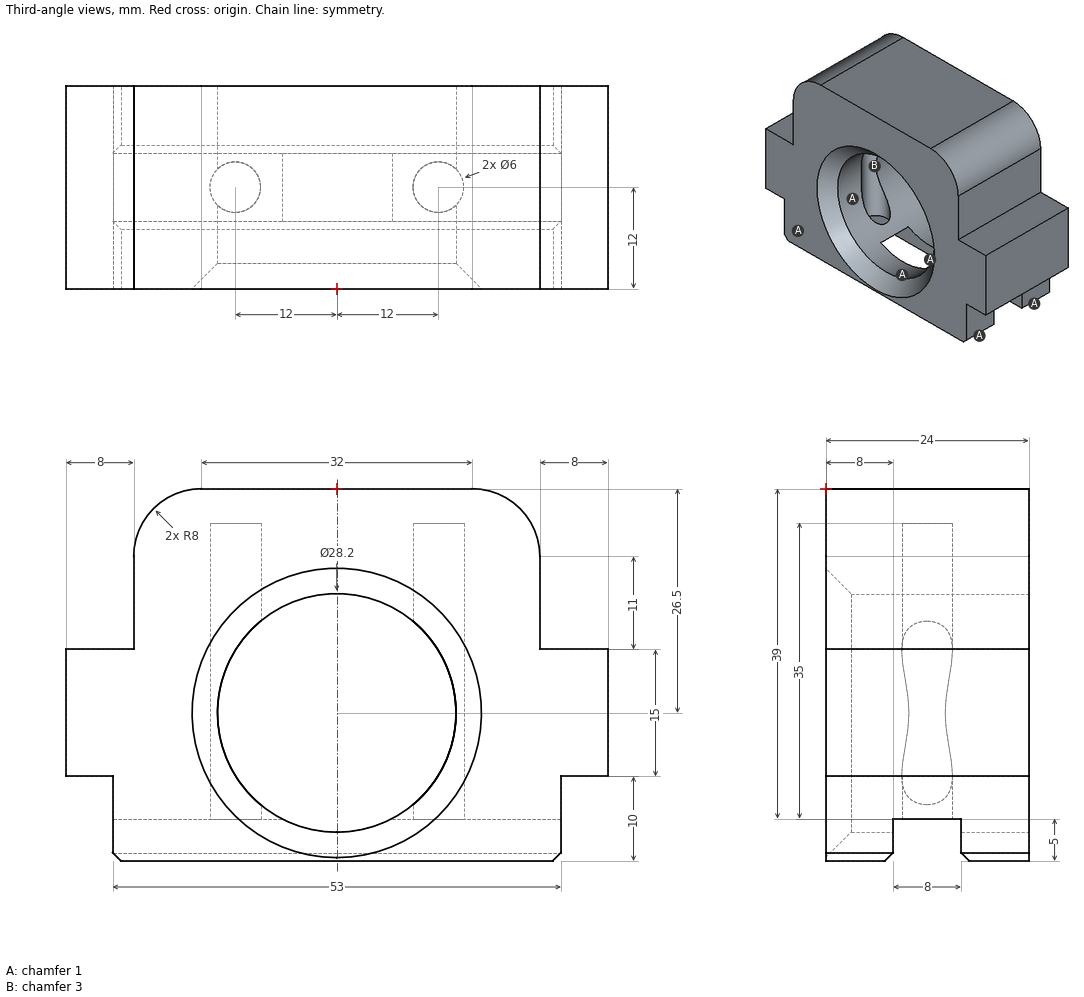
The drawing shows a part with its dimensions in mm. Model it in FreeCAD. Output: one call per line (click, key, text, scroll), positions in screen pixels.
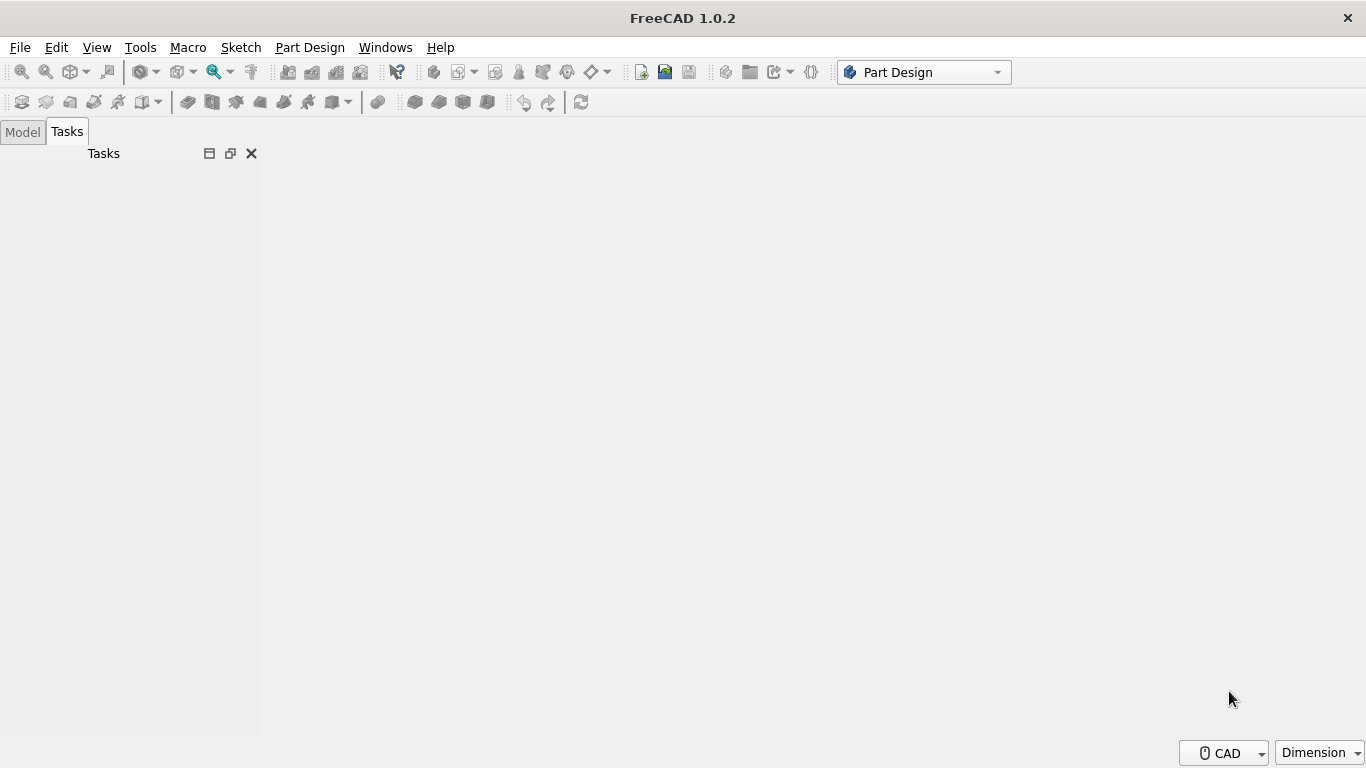
click(642, 72)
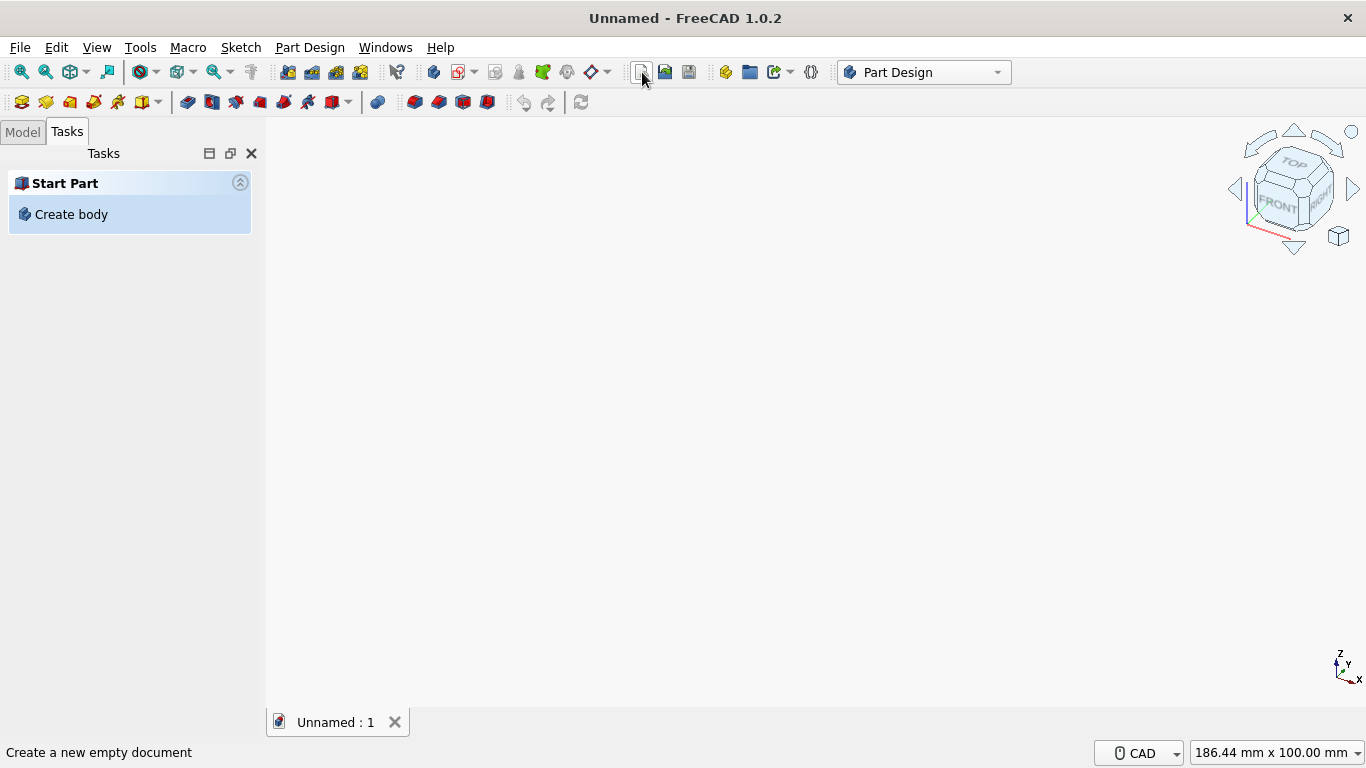
click(458, 72)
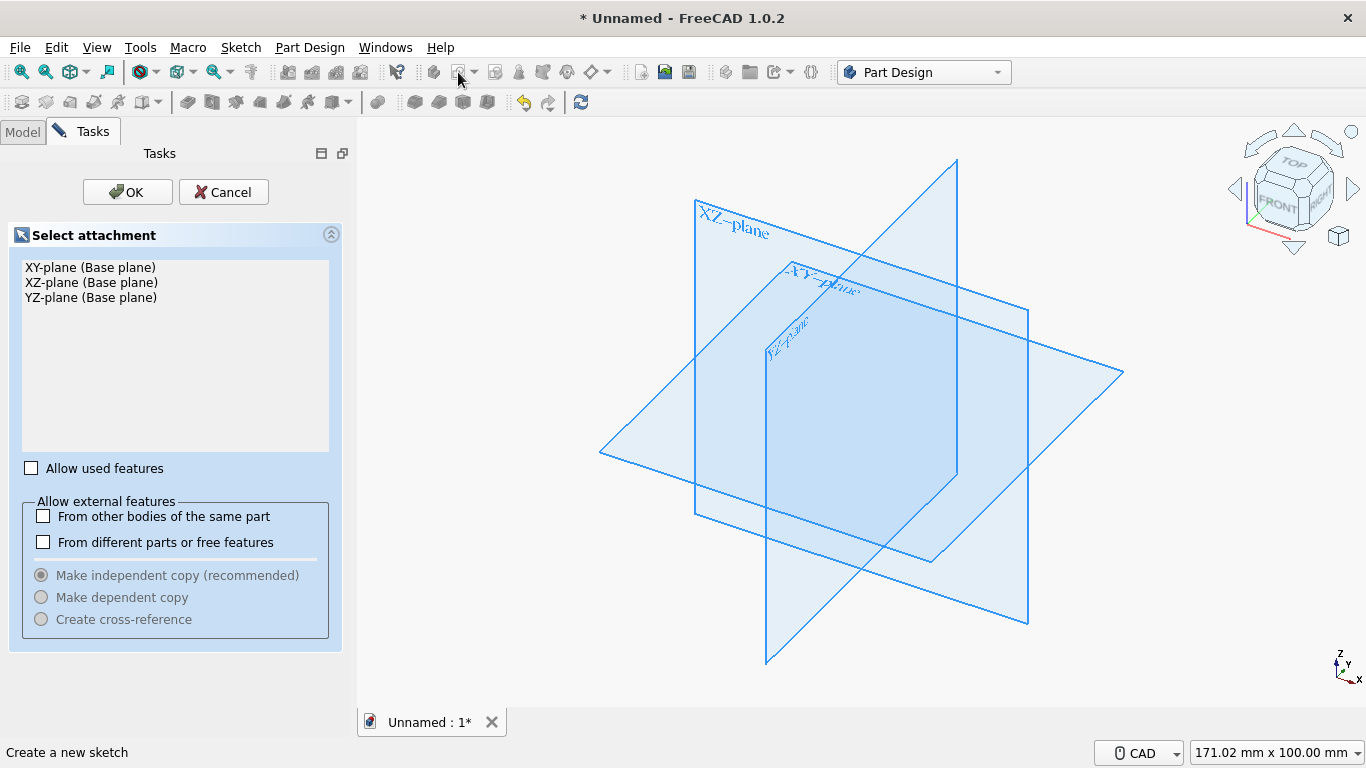
click(82, 282)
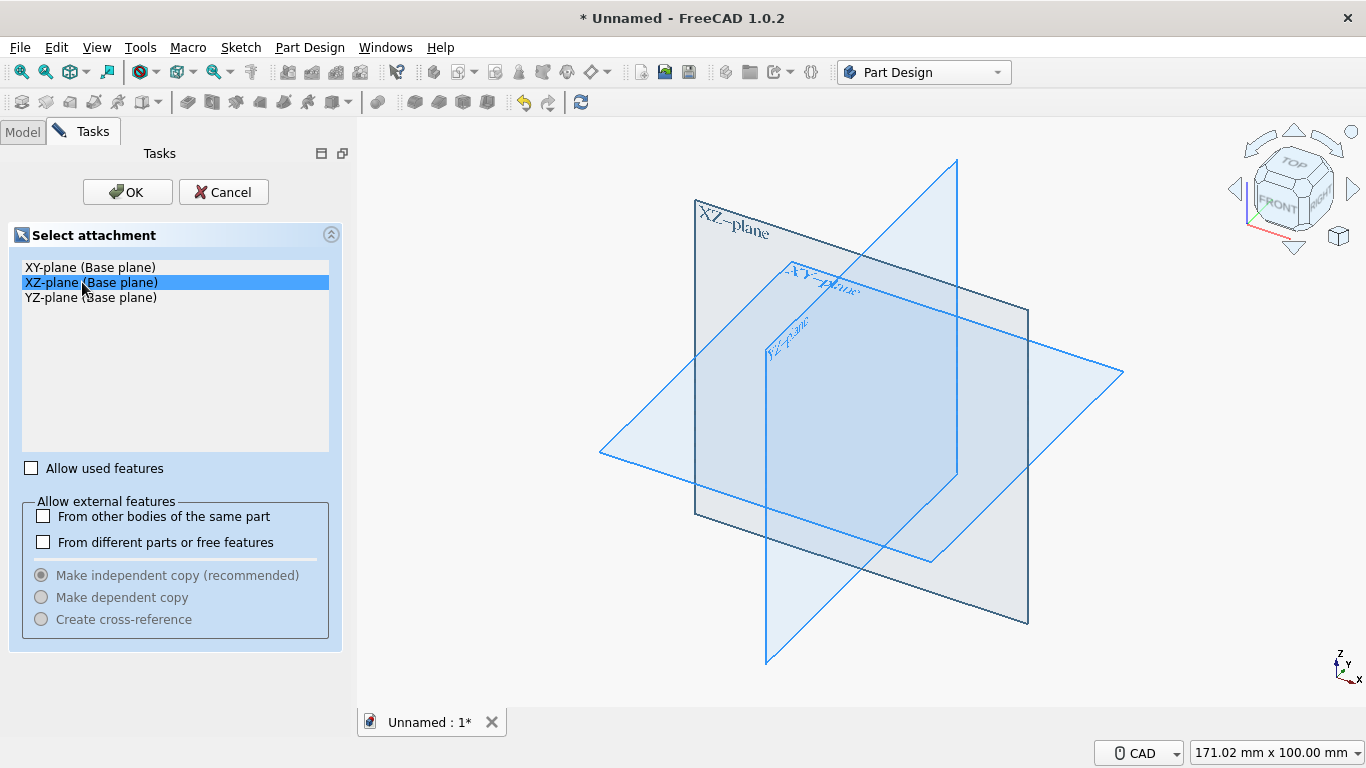
click(128, 192)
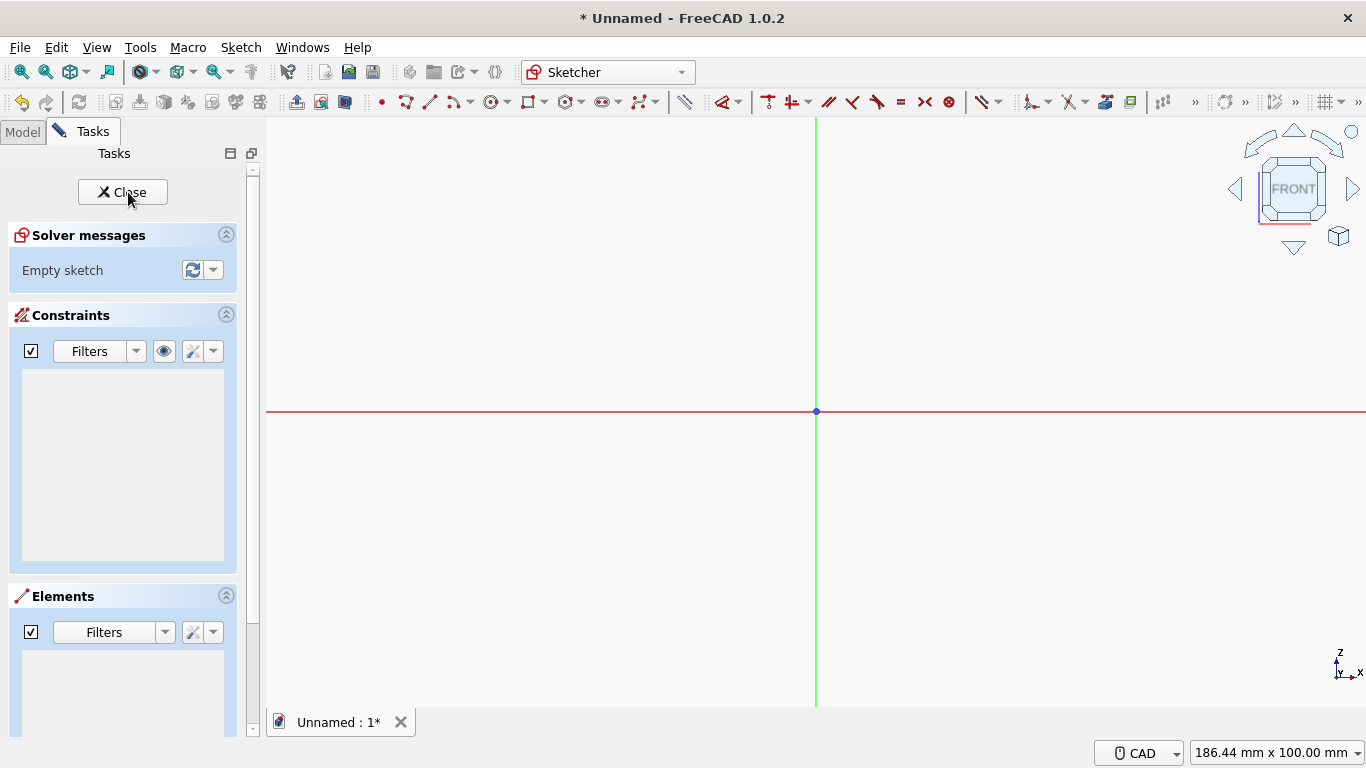
scroll(438, 145, down, 1)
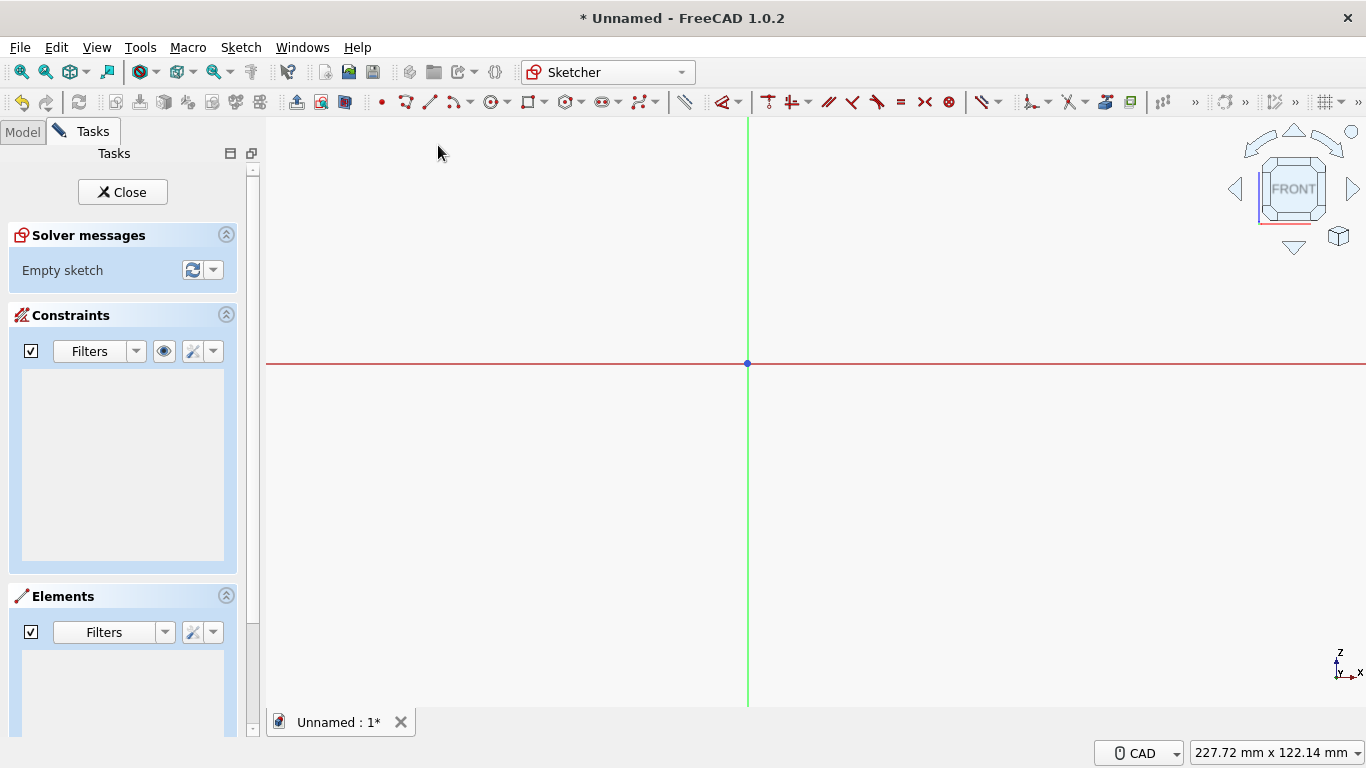
scroll(748, 540, up, 3)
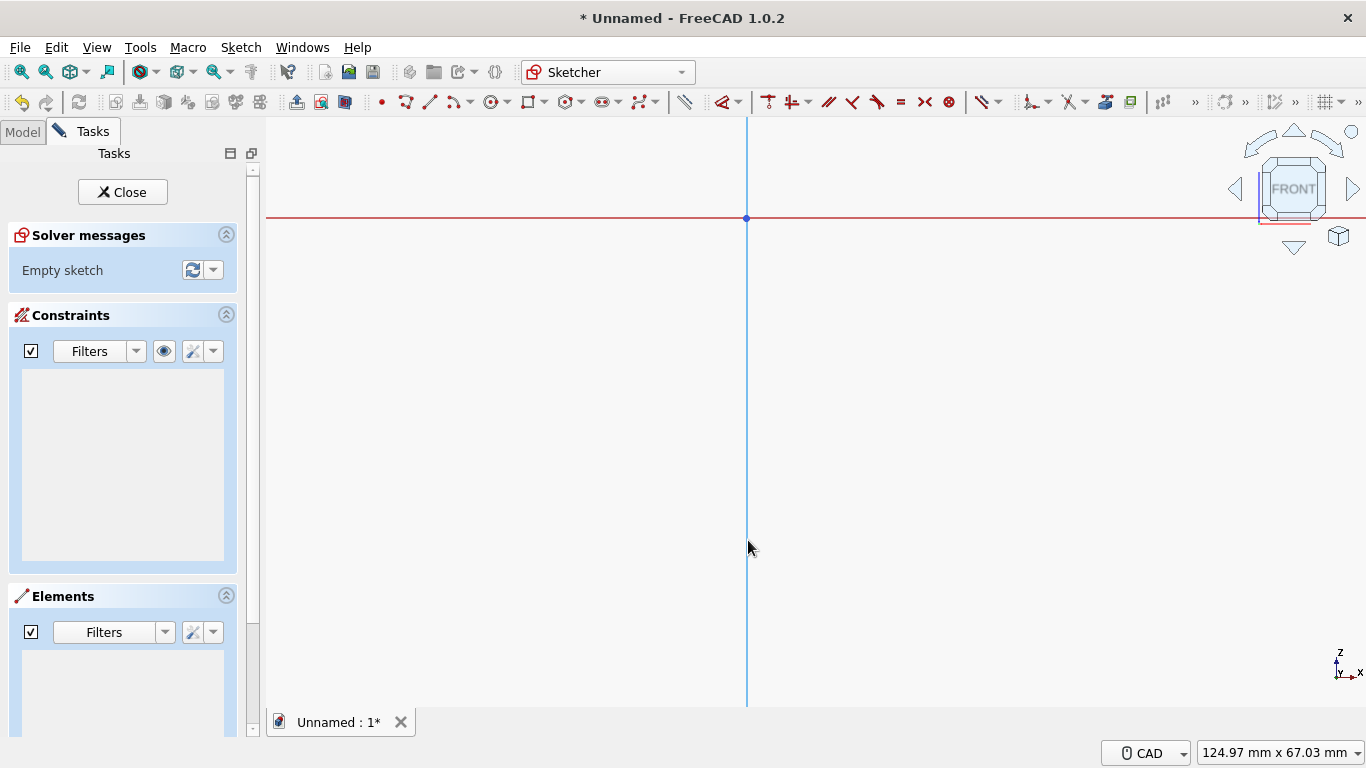
key(g)
key(l)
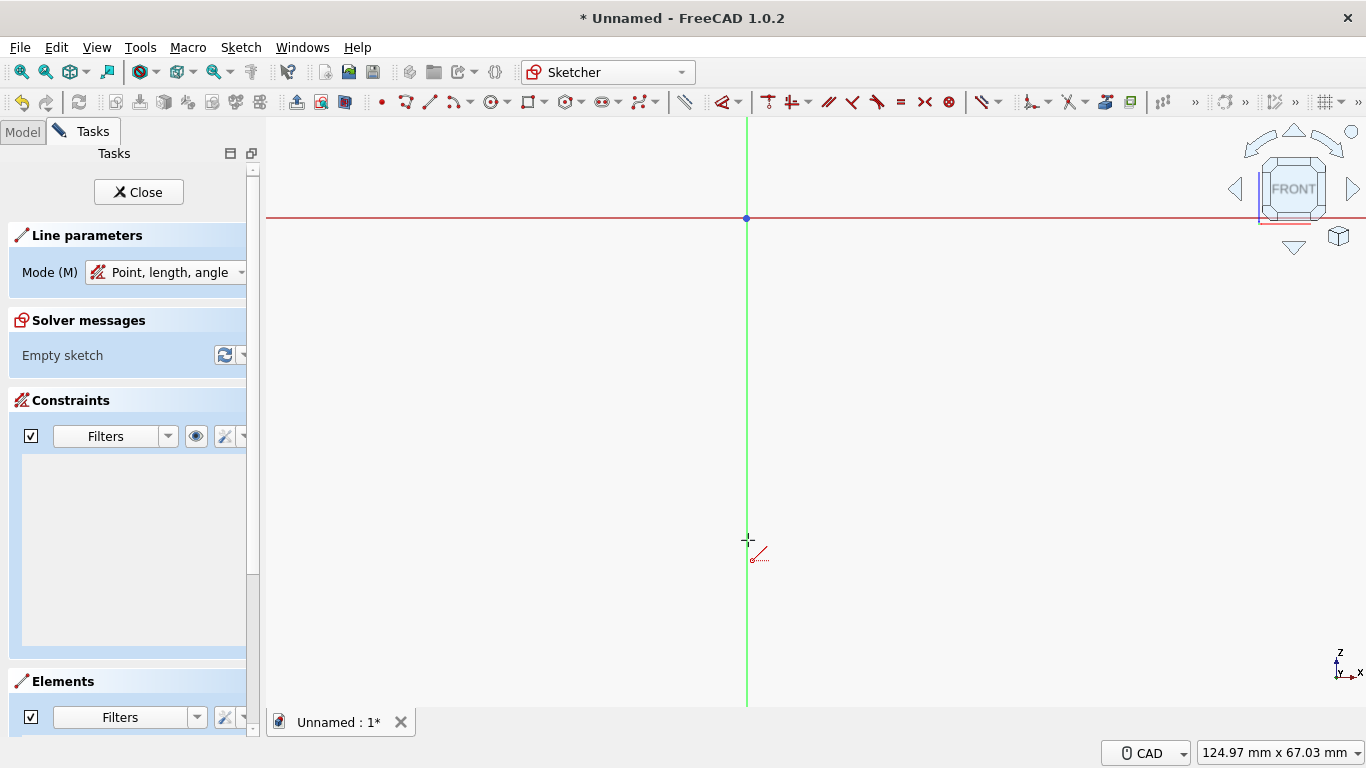
click(606, 218)
click(888, 227)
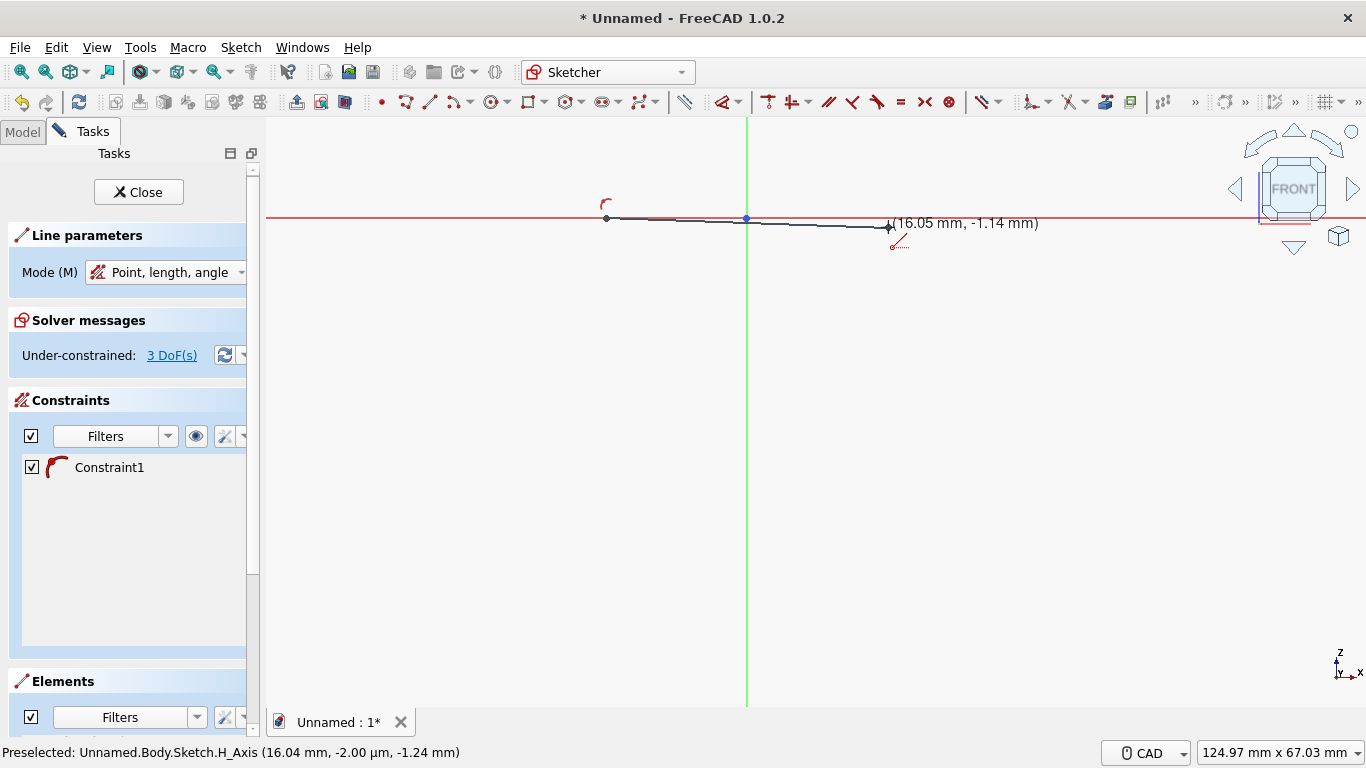
key(g)
key(m)